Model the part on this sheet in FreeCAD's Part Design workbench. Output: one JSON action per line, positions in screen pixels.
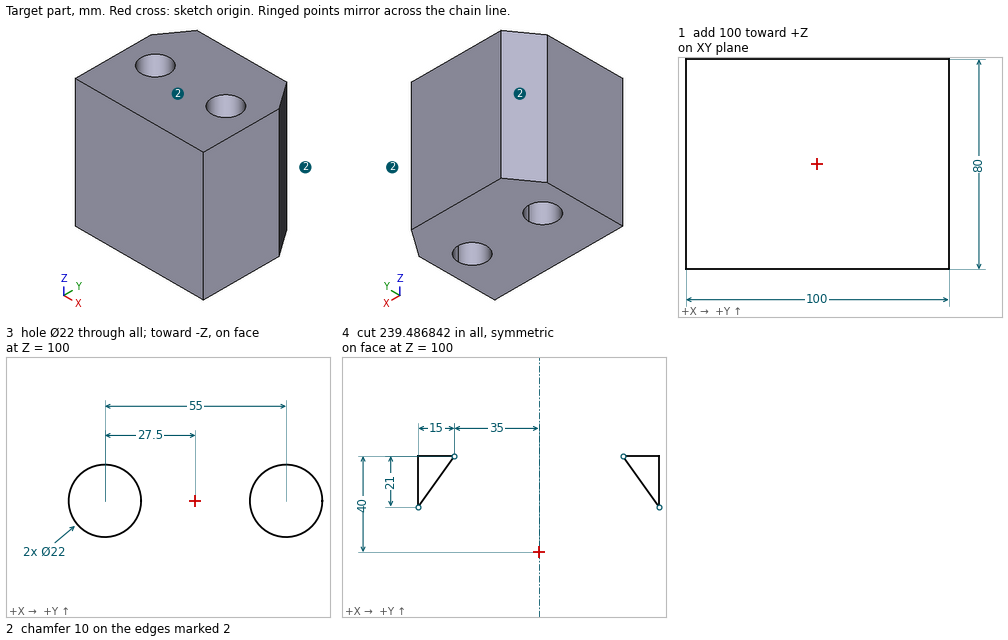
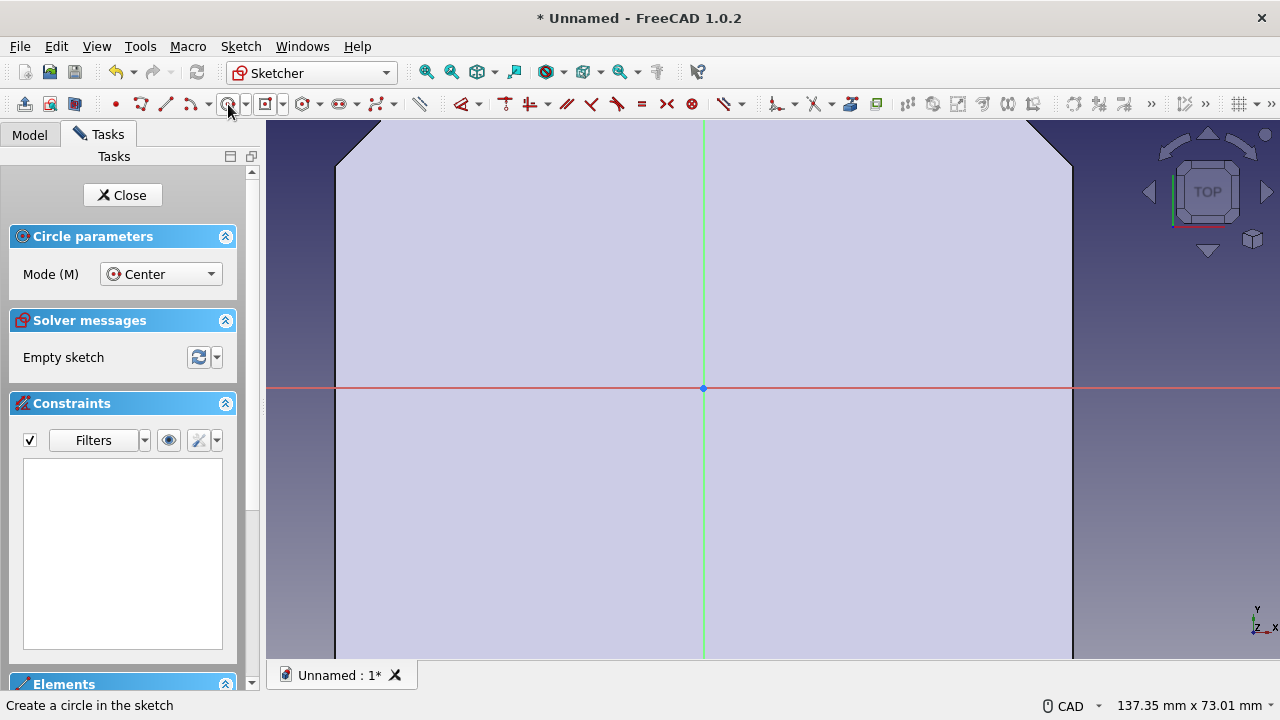
{"action": "left_click", "coordinate": [501, 388]}
{"action": "left_click", "coordinate": [558, 331]}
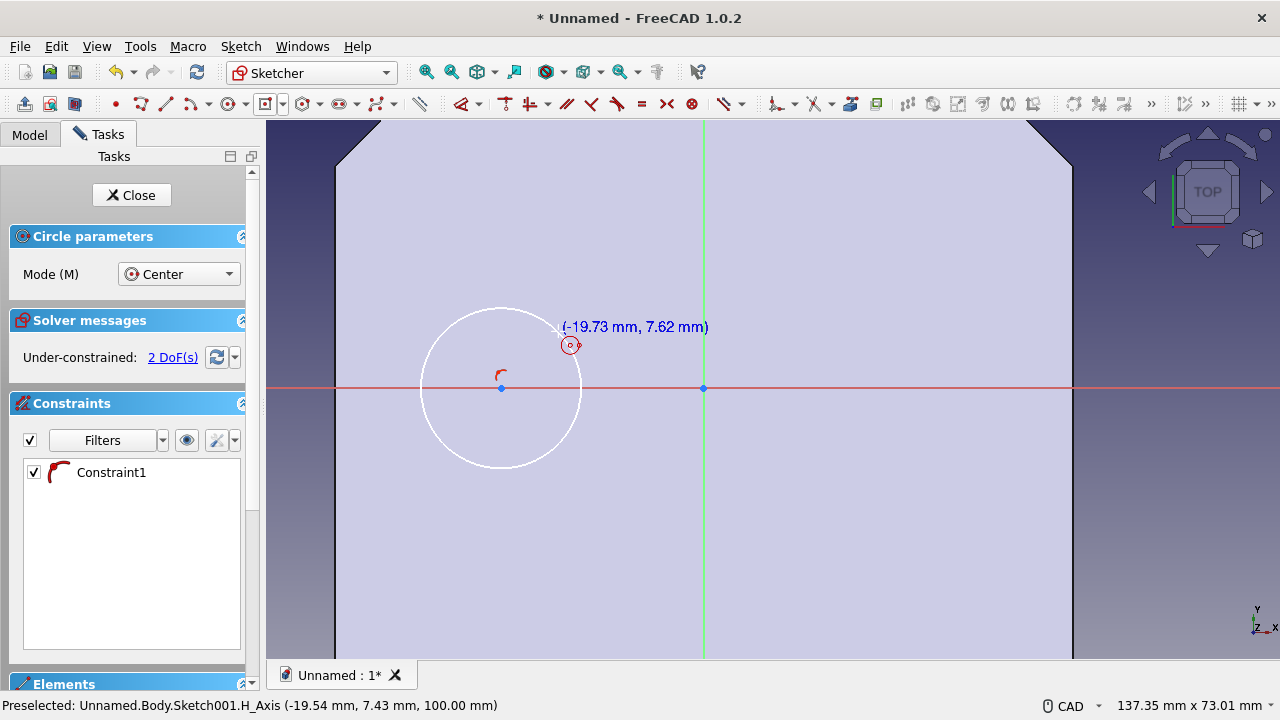
{"action": "left_click", "coordinate": [907, 388]}
{"action": "left_click", "coordinate": [964, 331]}
{"action": "key", "text": "Escape"}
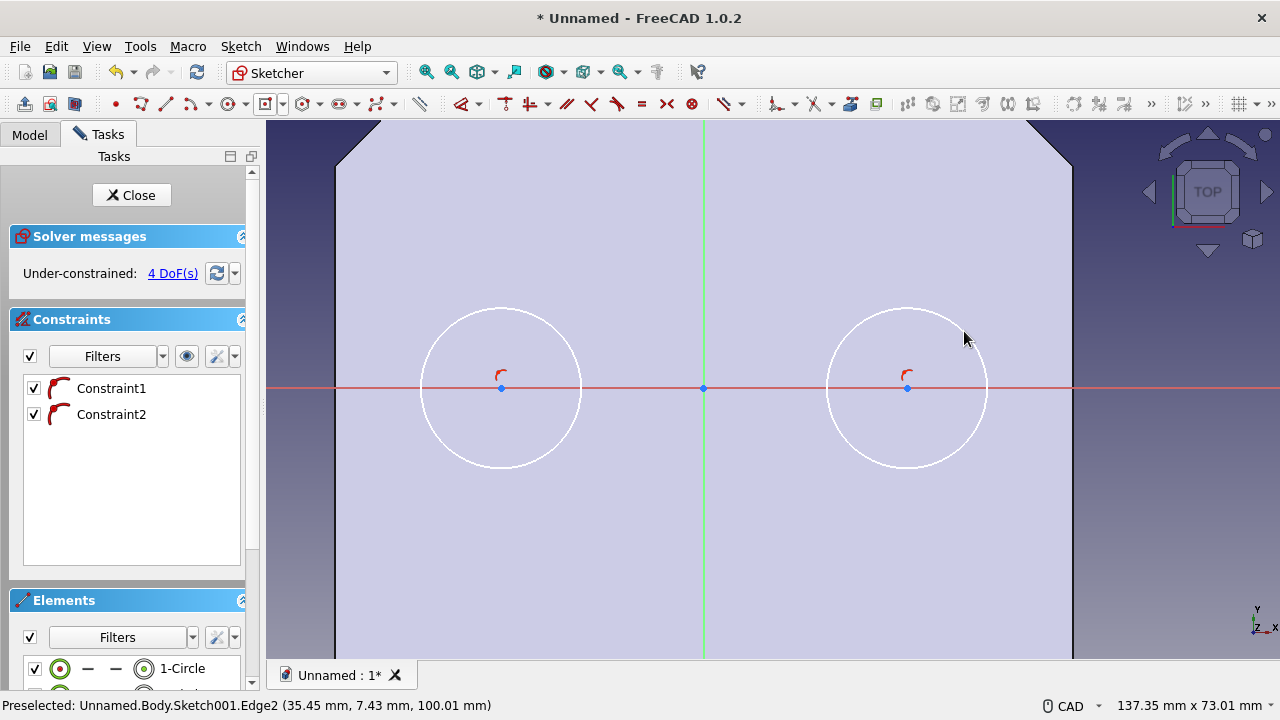
{"action": "left_click", "coordinate": [557, 331]}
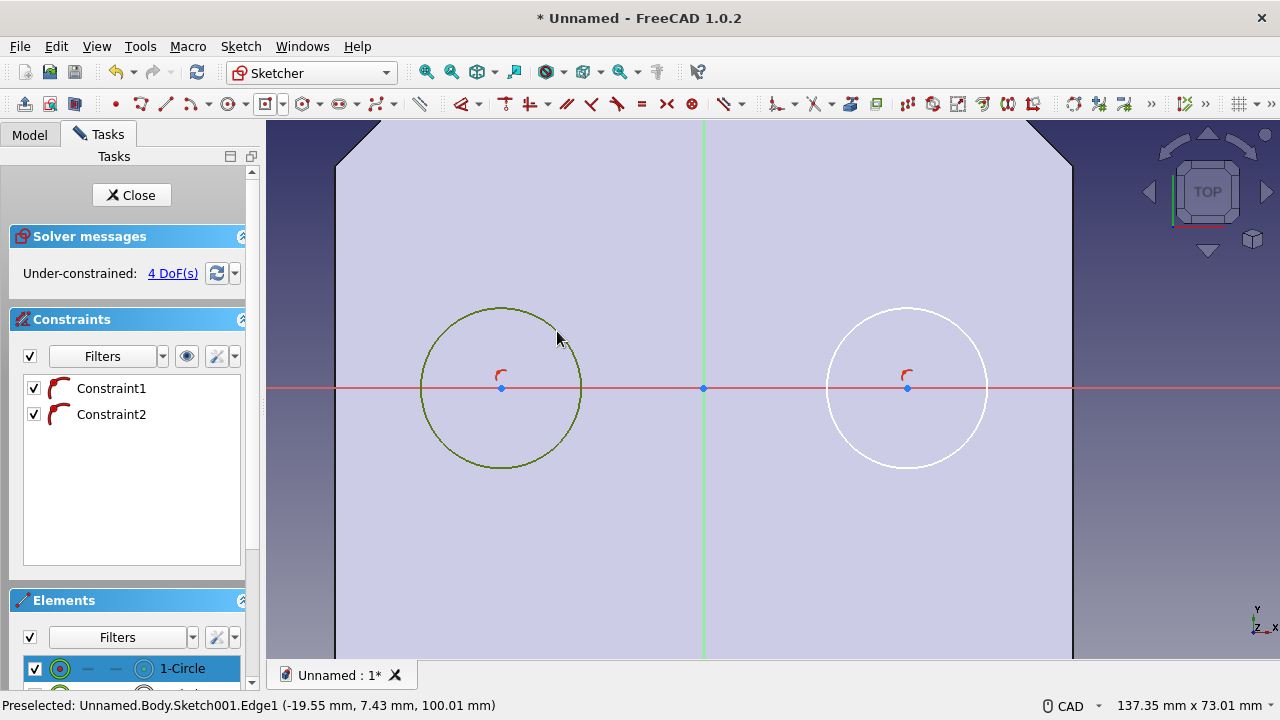
{"action": "left_click", "coordinate": [963, 331]}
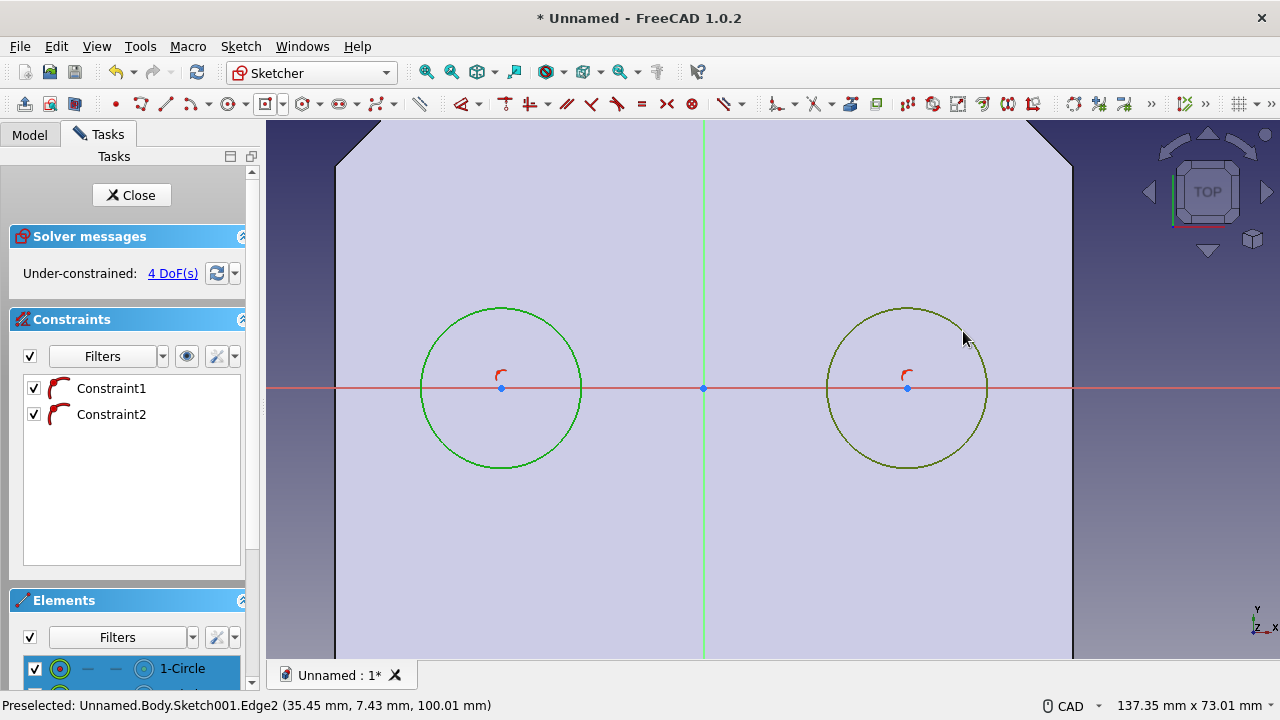
{"action": "left_click", "coordinate": [642, 104]}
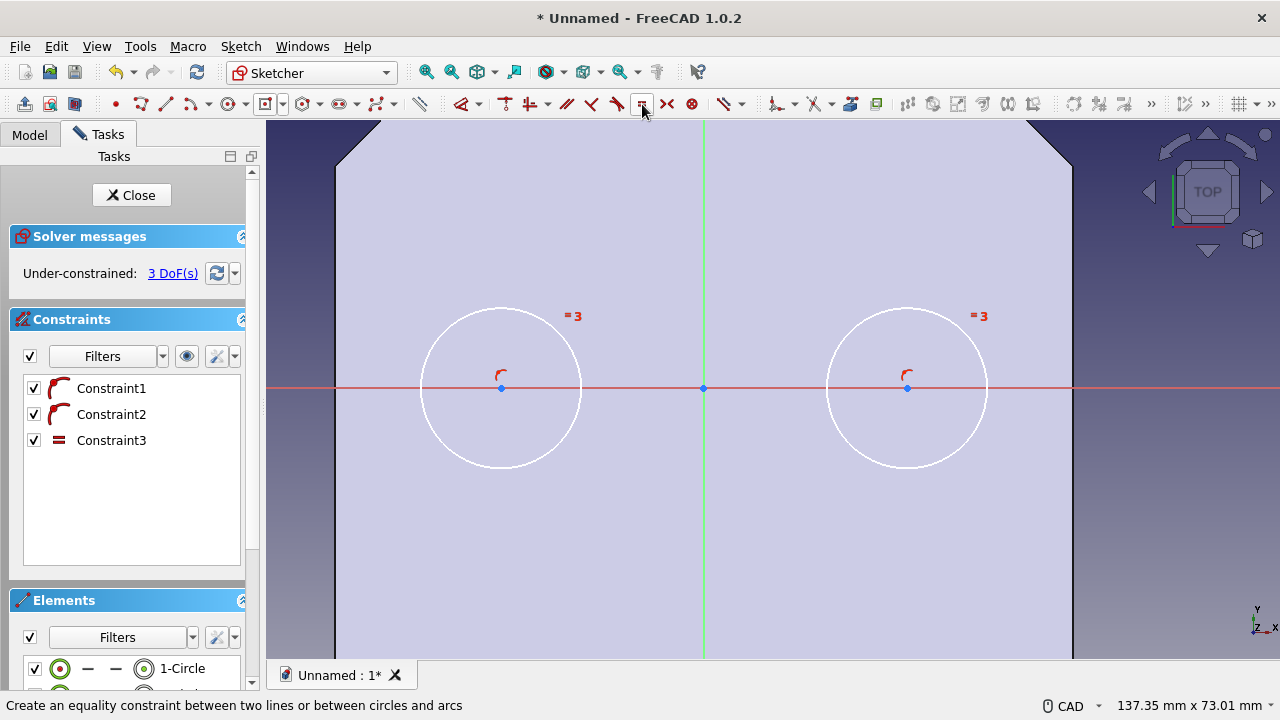
{"action": "left_click", "coordinate": [460, 104]}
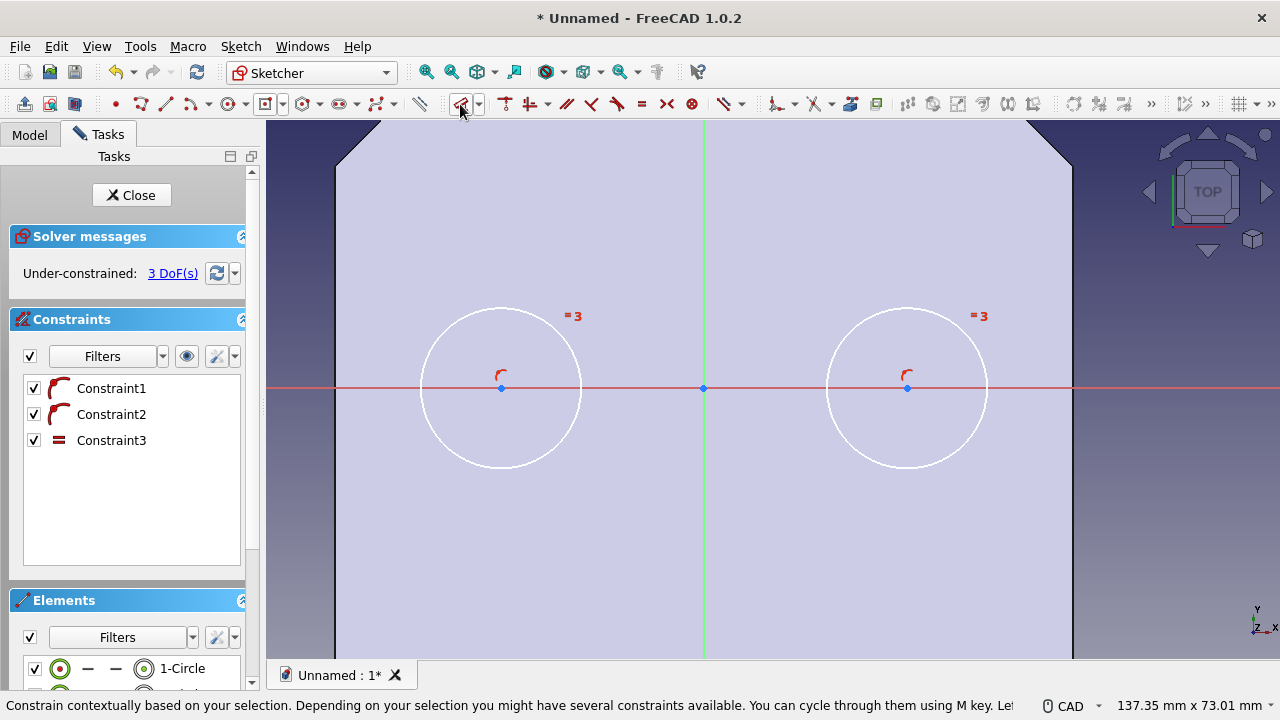
{"action": "left_click", "coordinate": [557, 331]}
{"action": "left_click", "coordinate": [579, 308]}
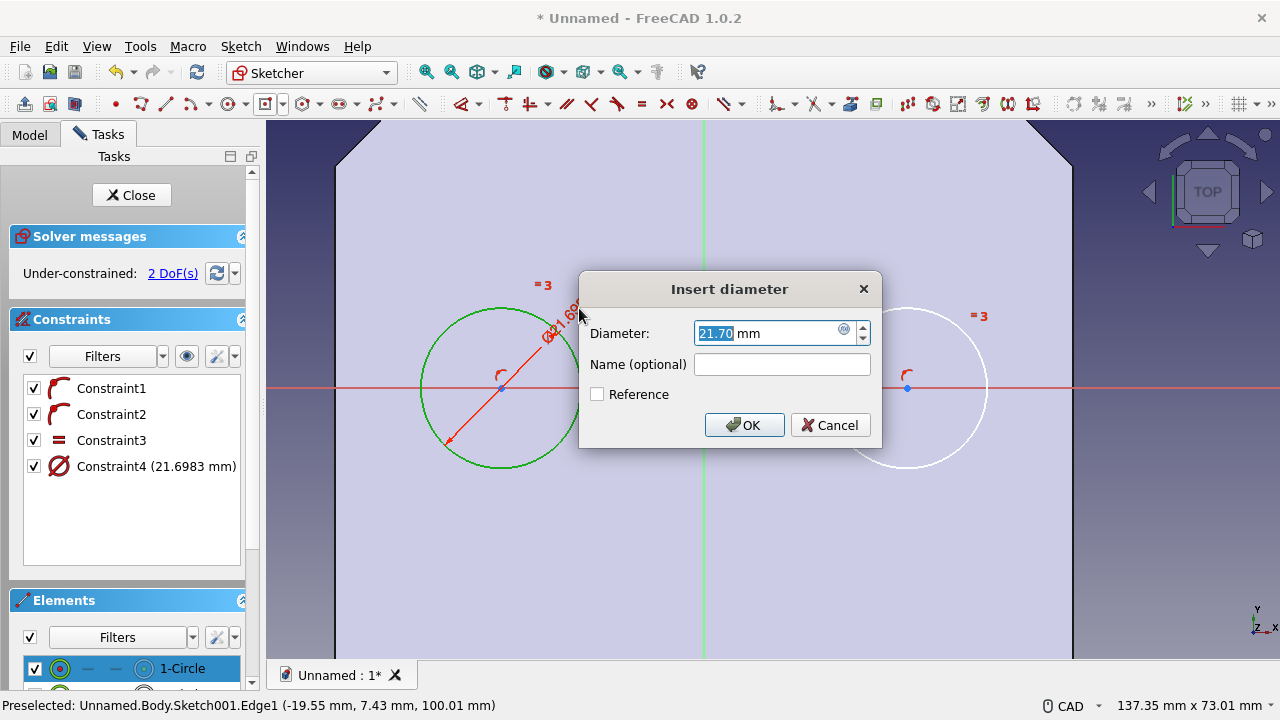
{"action": "type", "text": "22"}
{"action": "key", "text": "Return"}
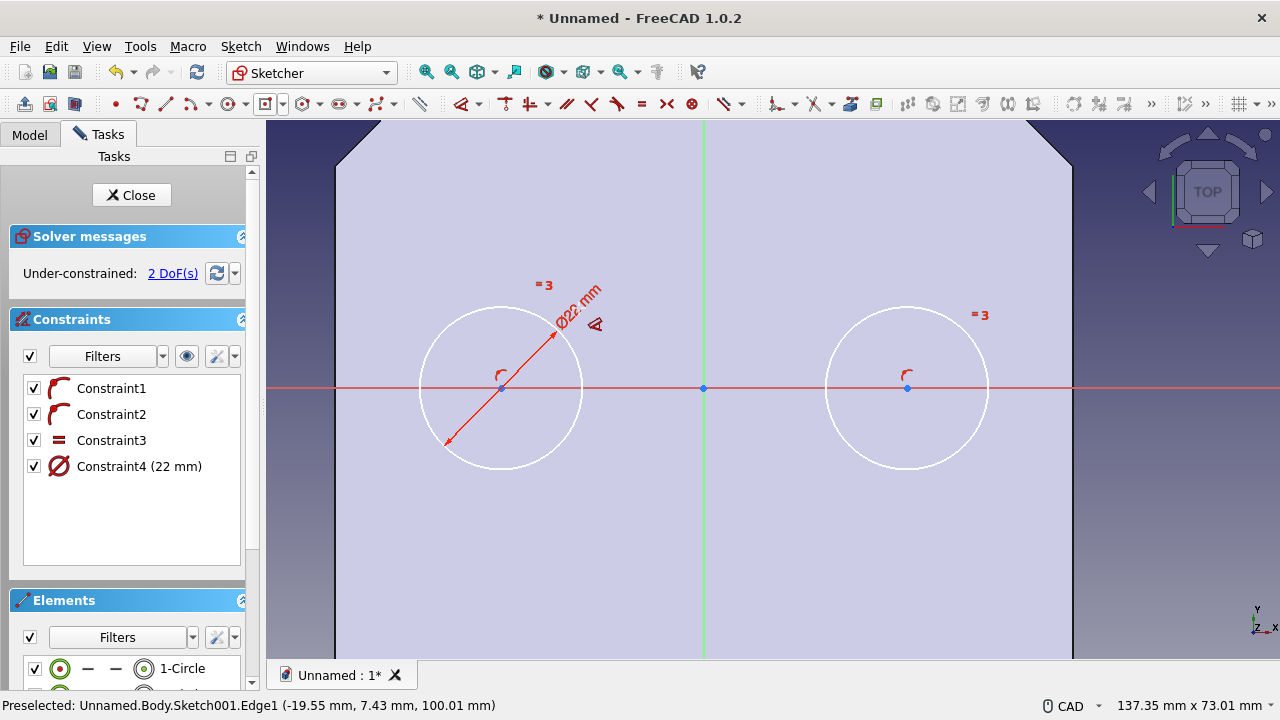
{"action": "left_click", "coordinate": [501, 388]}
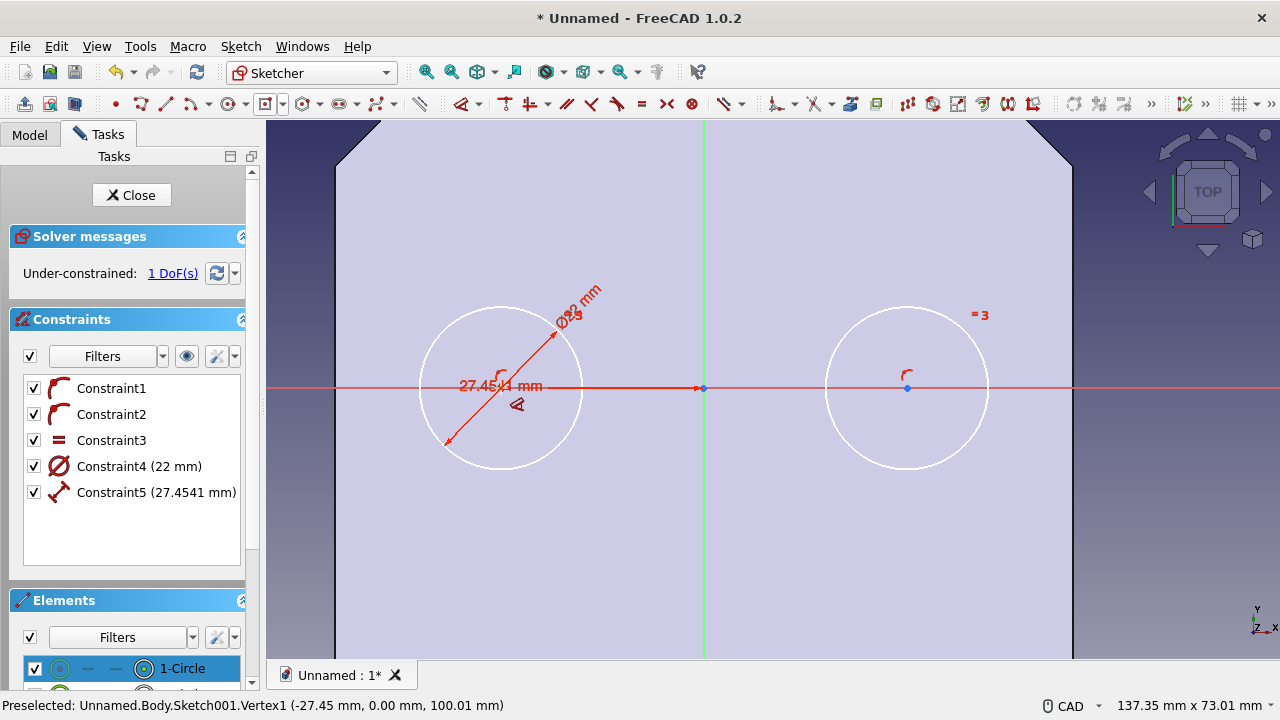
{"action": "left_click", "coordinate": [907, 388]}
{"action": "left_click", "coordinate": [611, 422]}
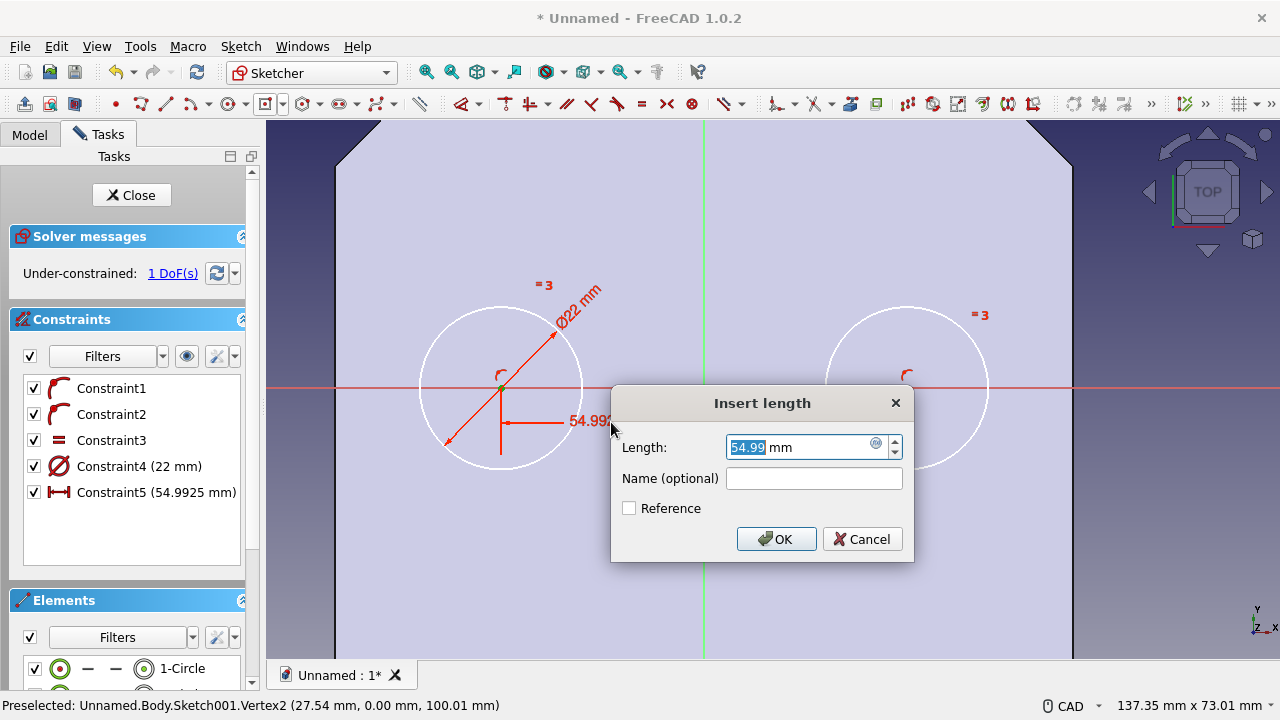
{"action": "type", "text": "55"}
{"action": "key", "text": "Return"}